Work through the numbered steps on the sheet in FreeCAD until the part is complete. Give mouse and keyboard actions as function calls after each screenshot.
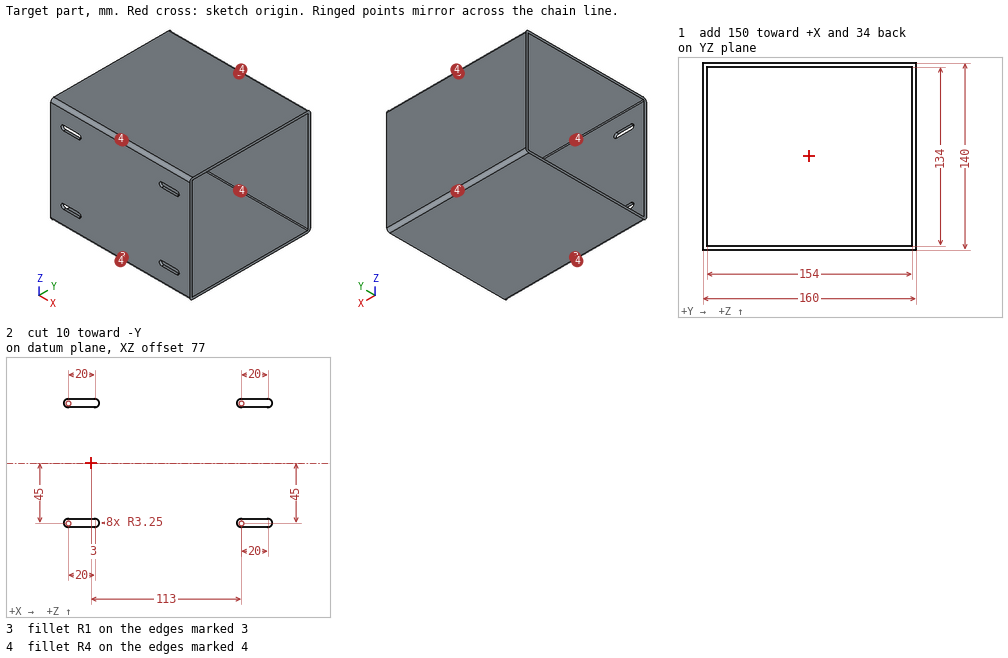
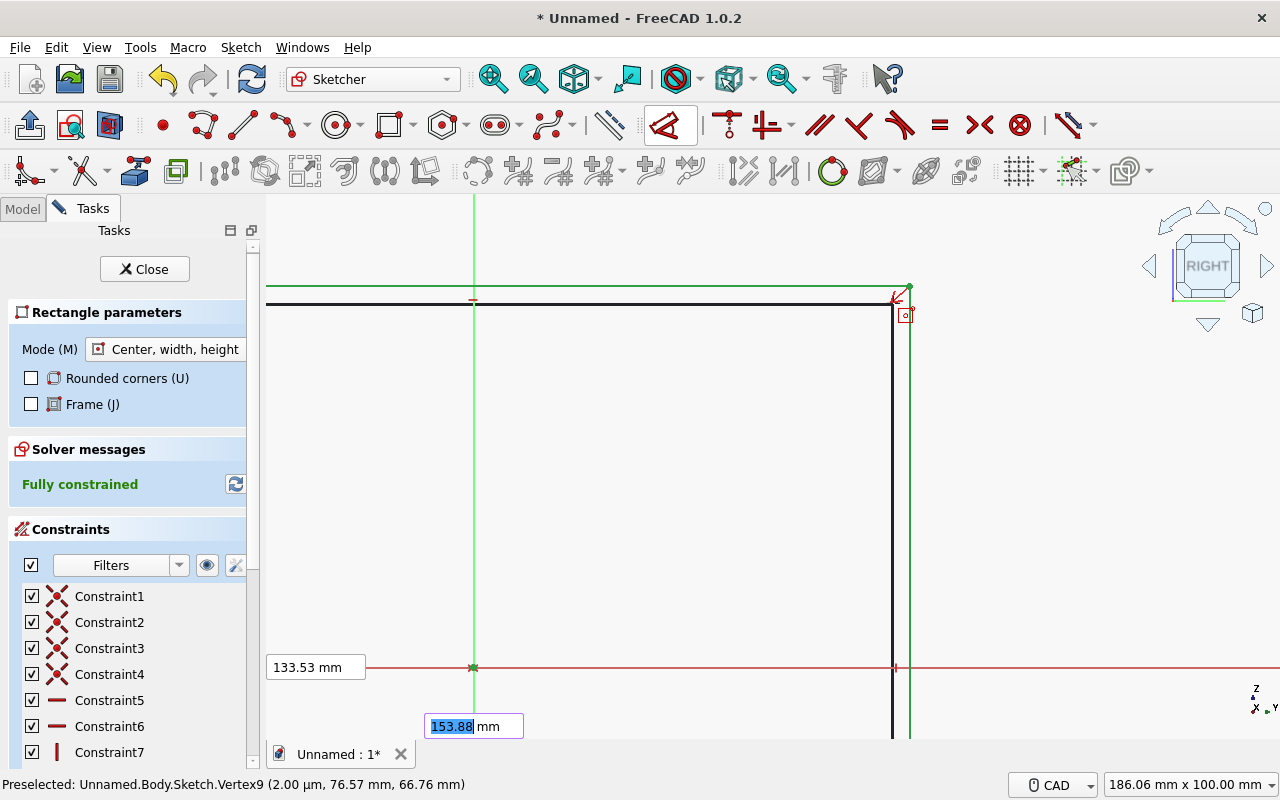
text(154)
key(Tab)
text(134)
key(Return)
key(Escape)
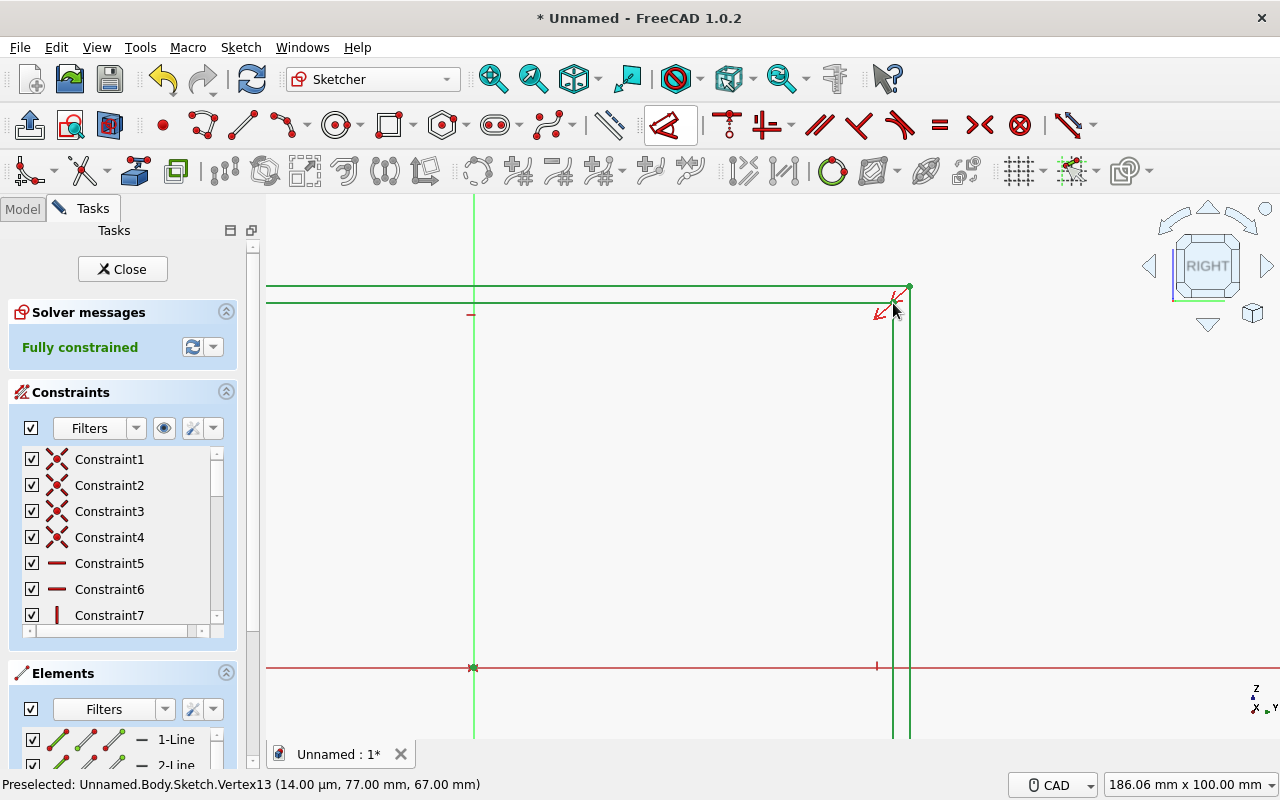
click(123, 269)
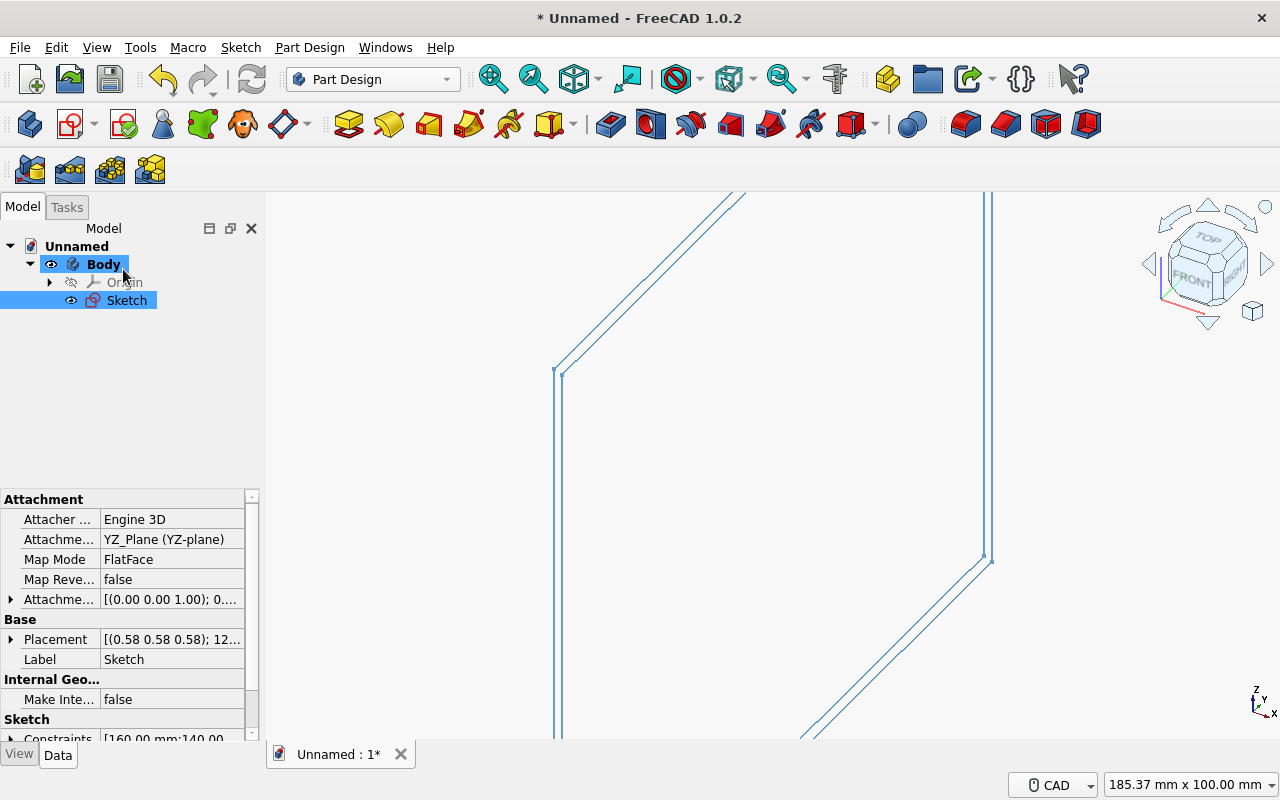
click(350, 124)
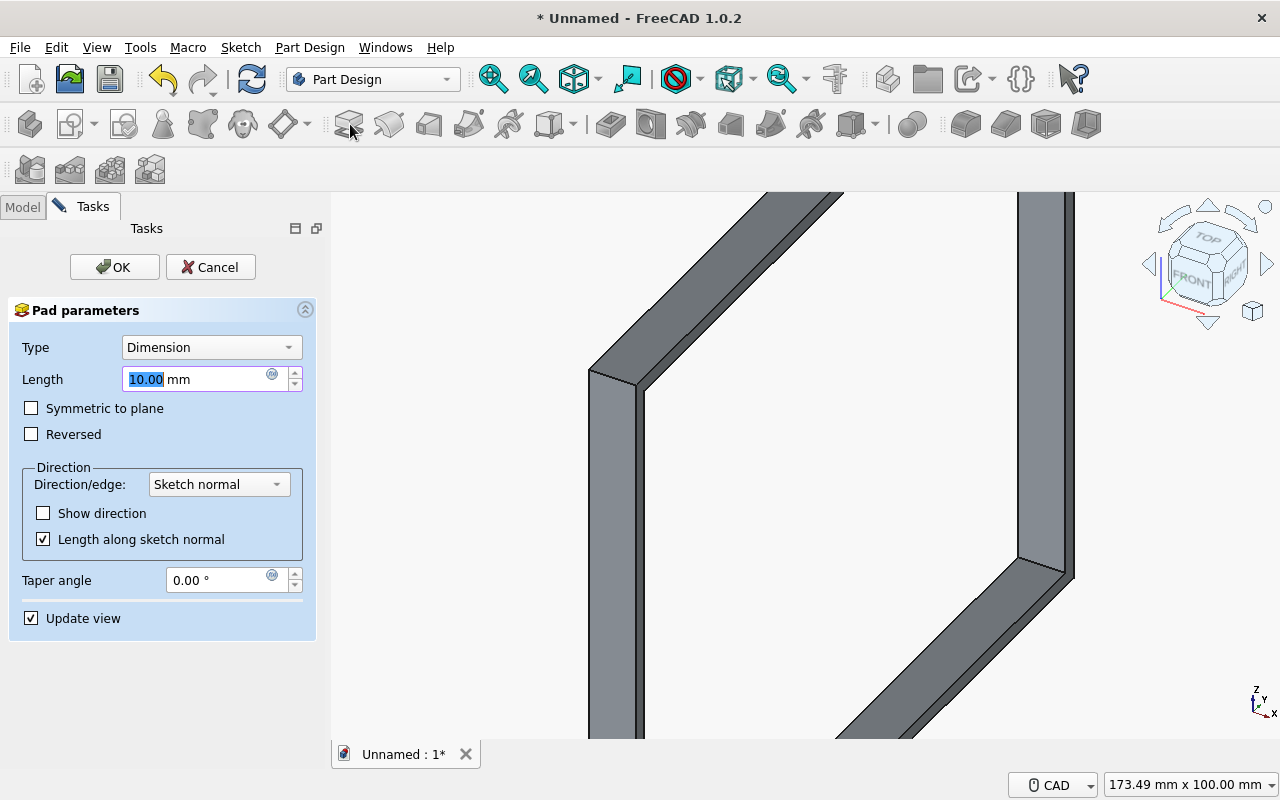
click(212, 348)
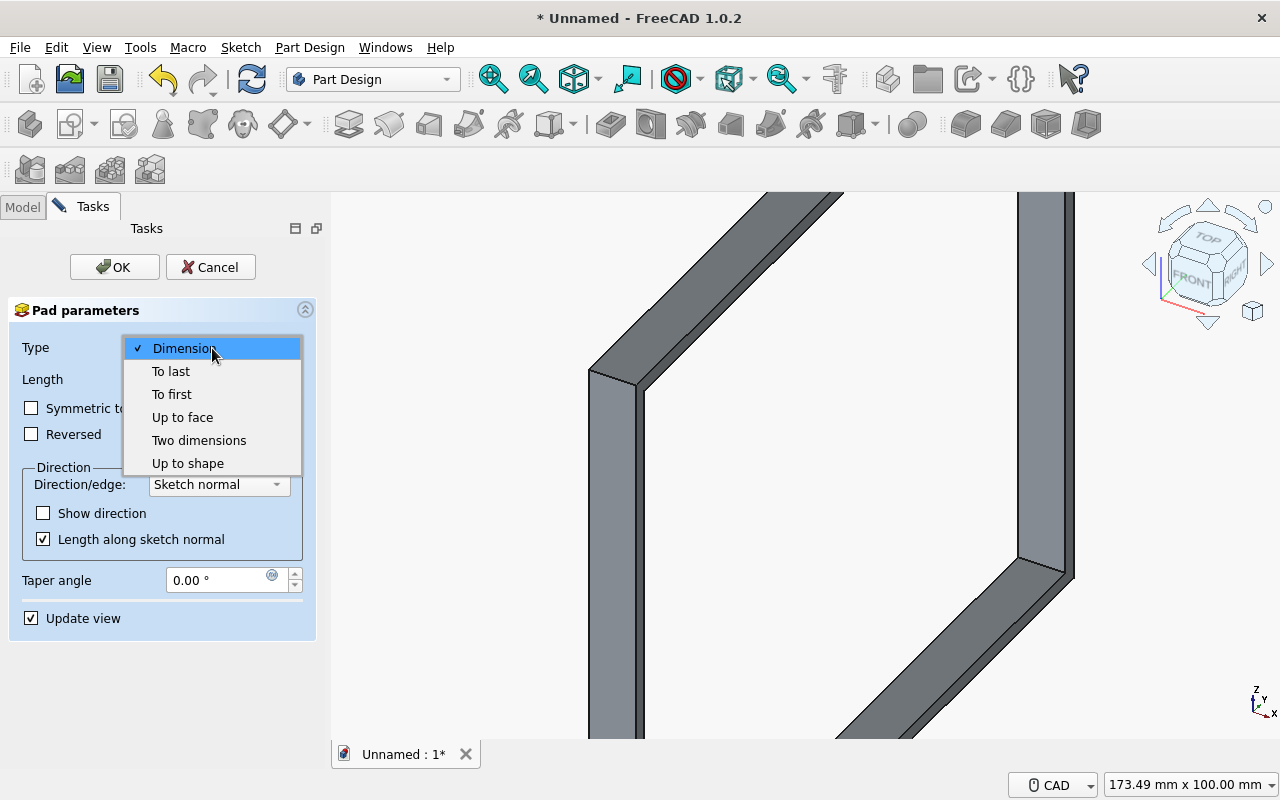
click(212, 440)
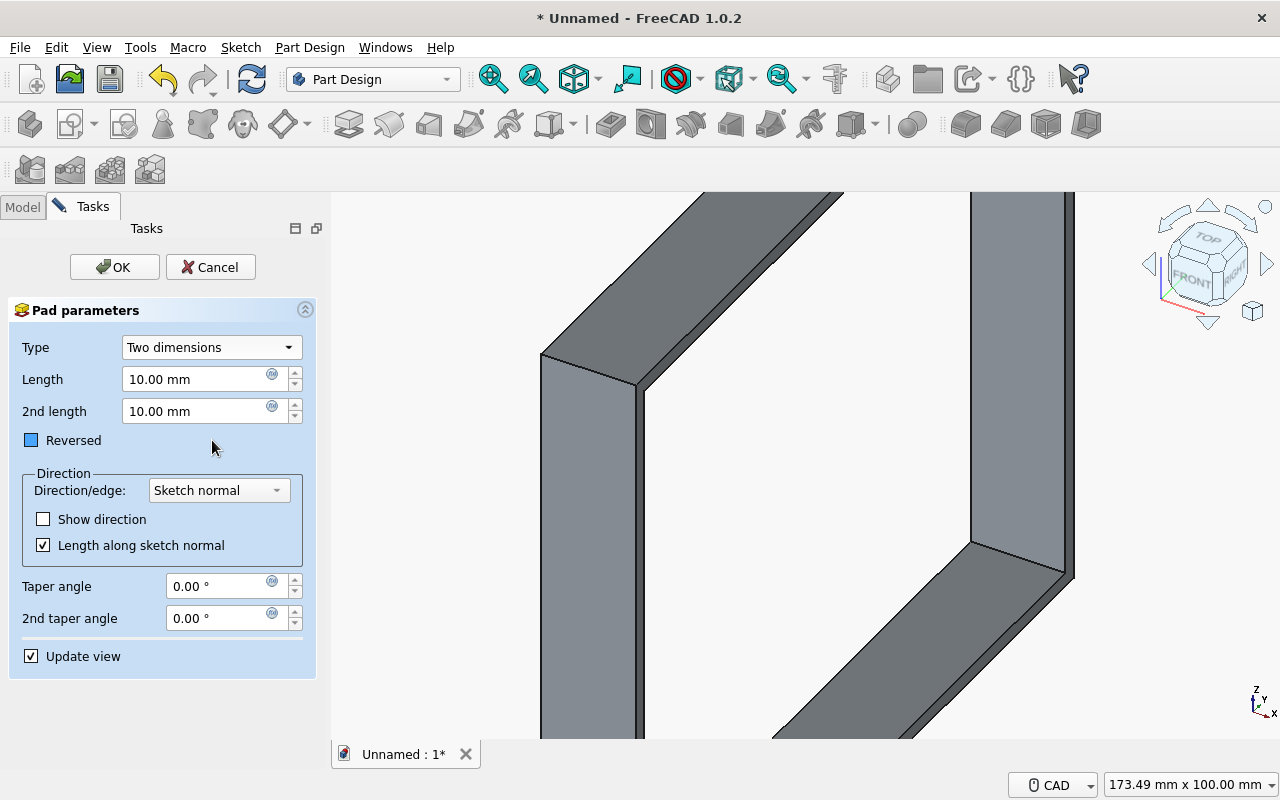
triple_click(204, 379)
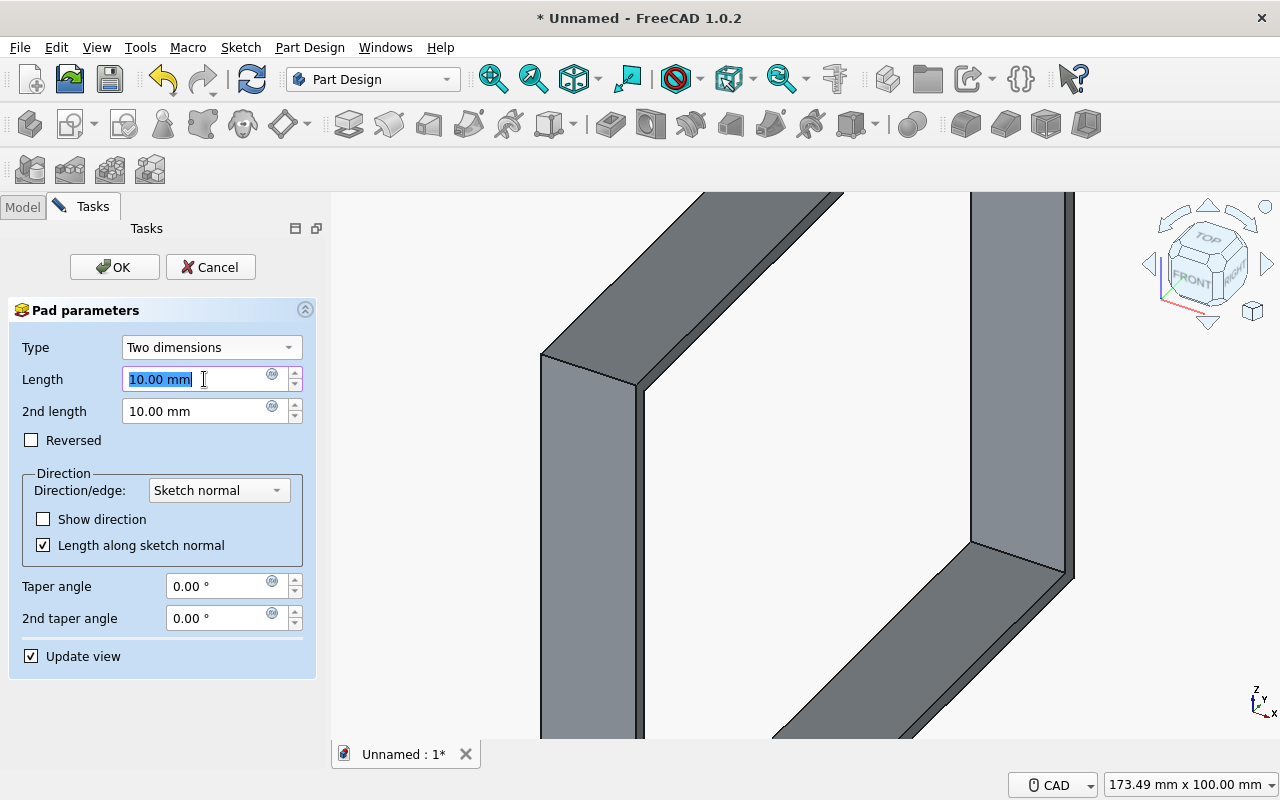
text(150)
key(Tab)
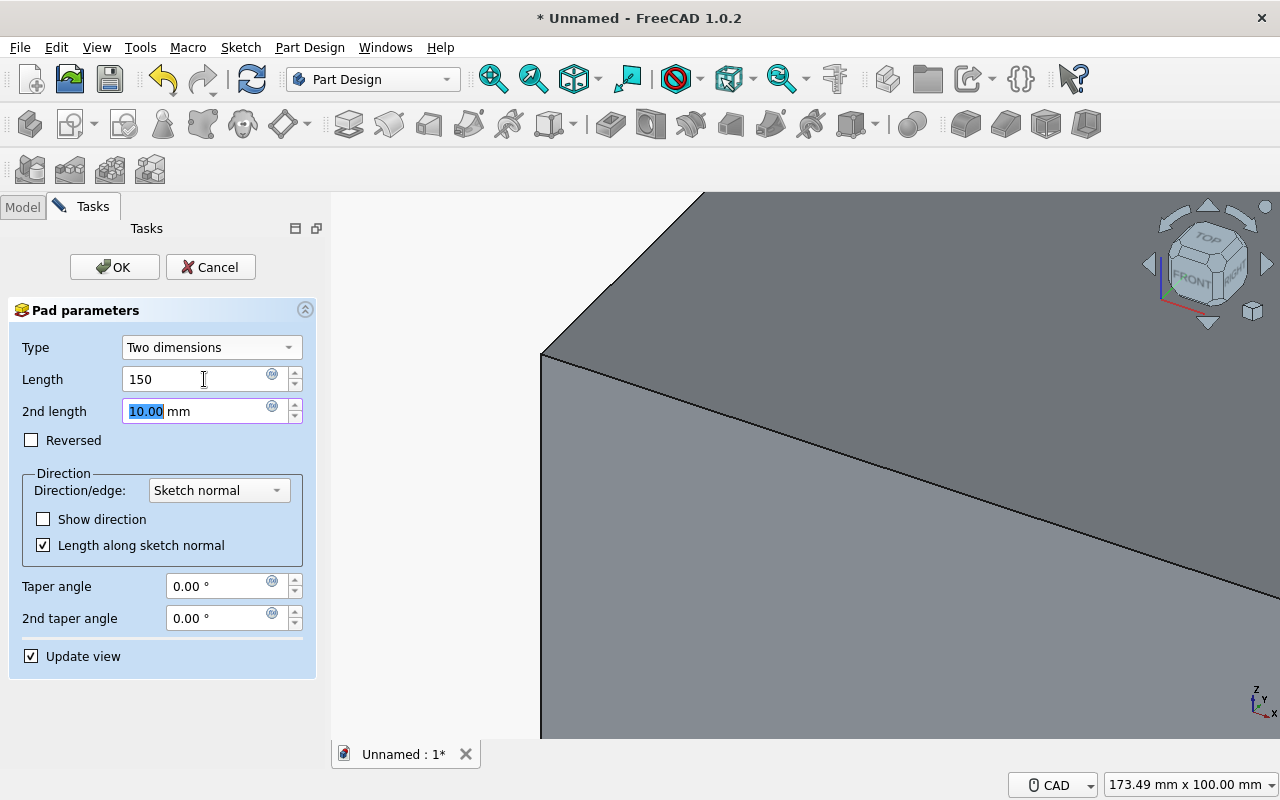
text(34)
key(Tab)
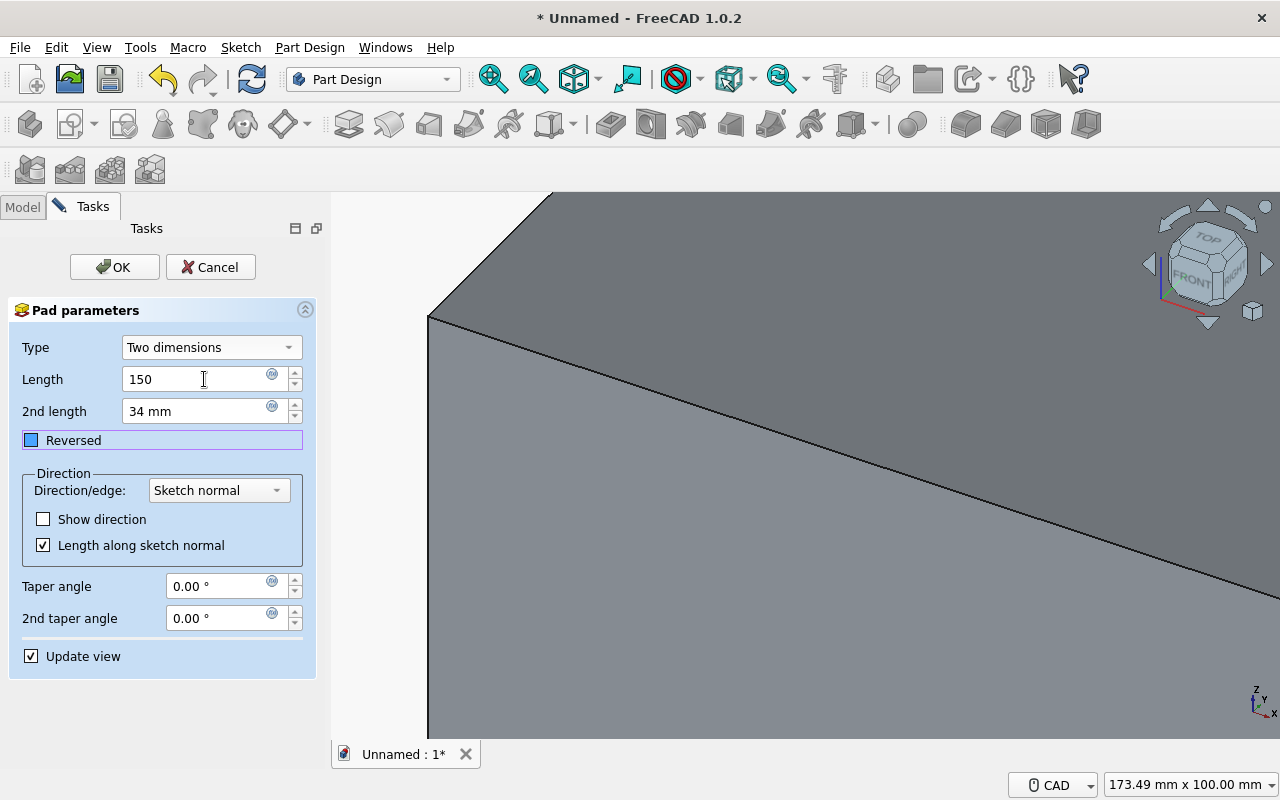
click(115, 267)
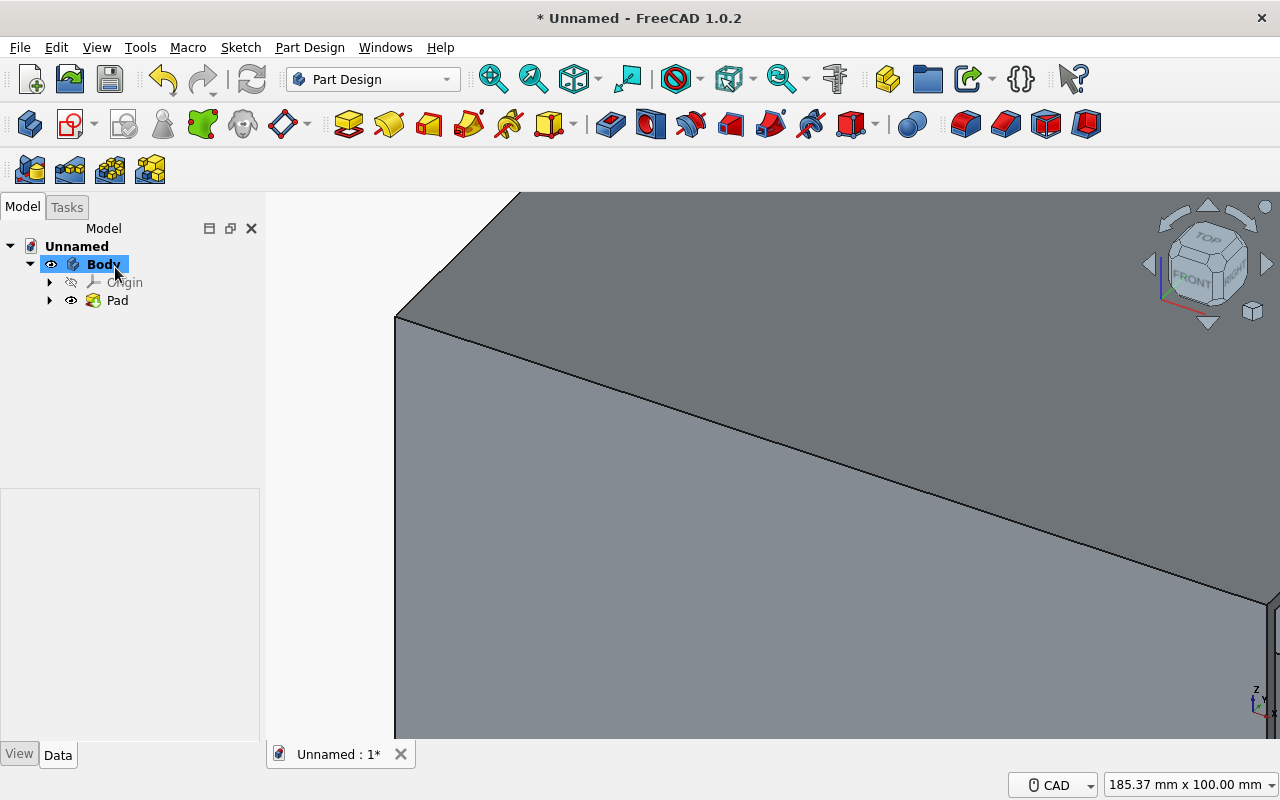
key(v)
key(f)